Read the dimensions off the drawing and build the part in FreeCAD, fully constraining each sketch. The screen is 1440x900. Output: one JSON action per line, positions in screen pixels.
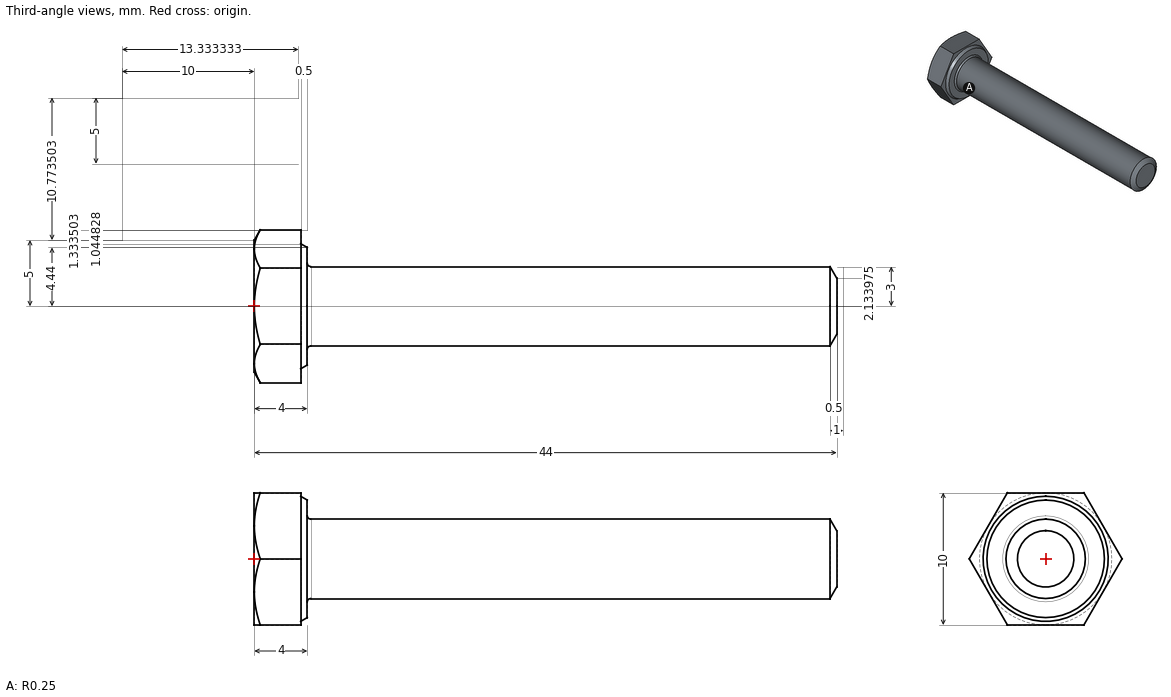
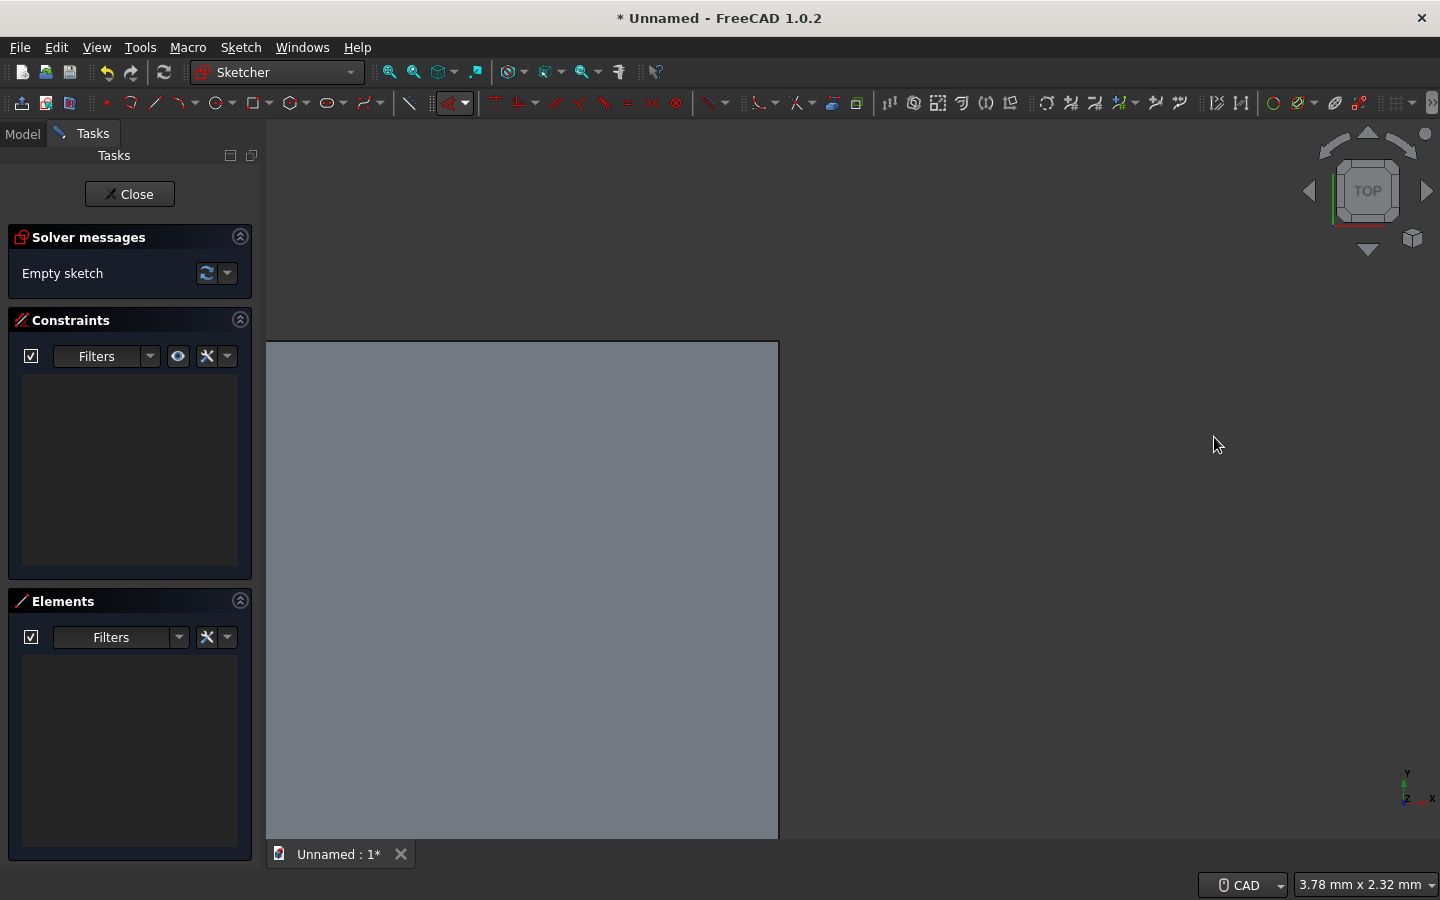
{"action": "scroll", "coordinate": [771, 470], "scroll_direction": "up", "scroll_amount": 3}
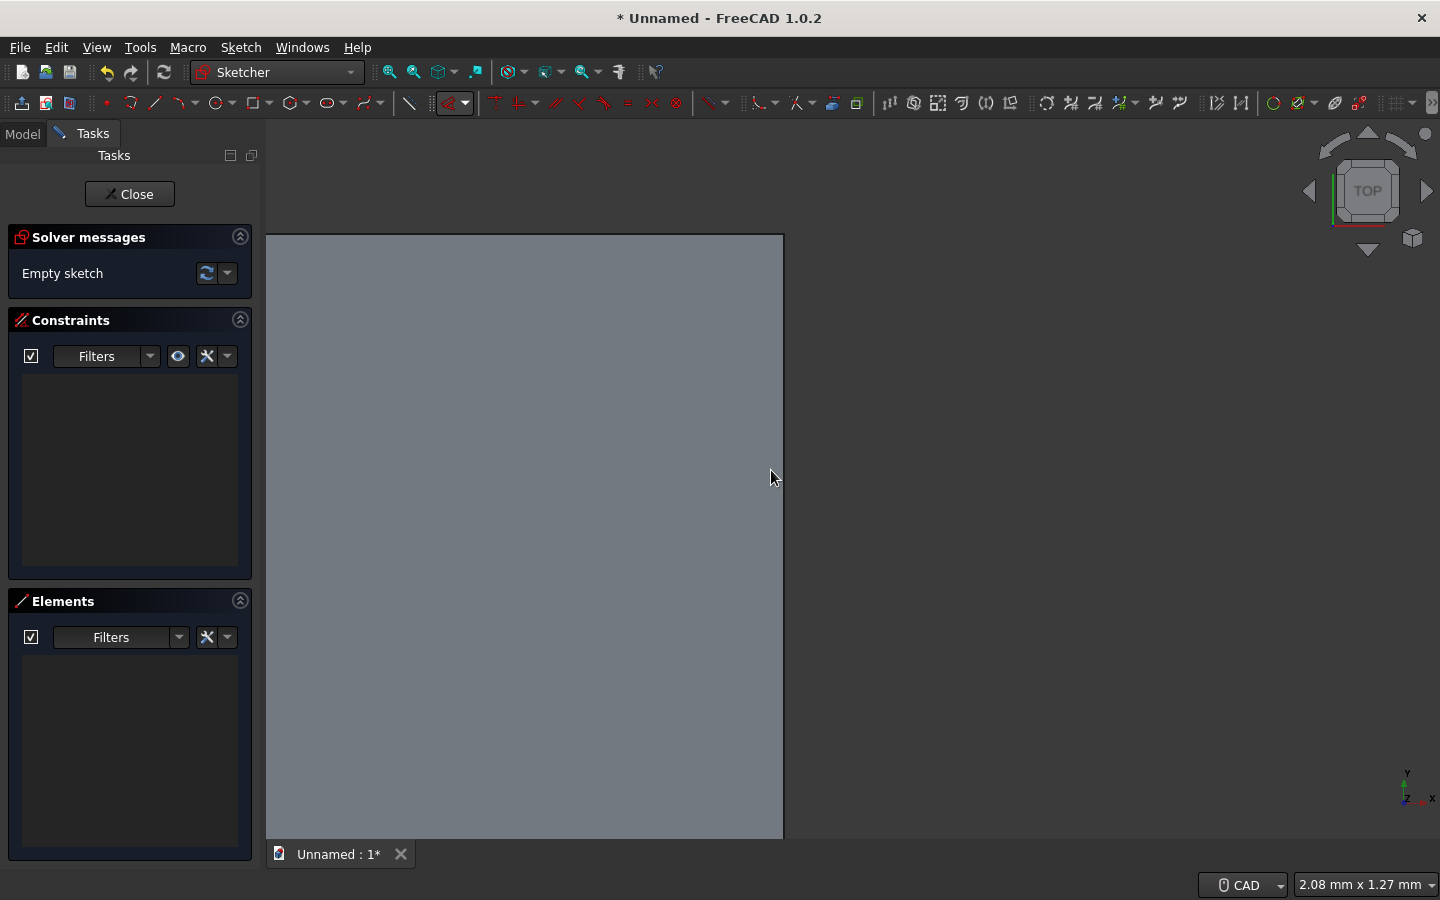
{"action": "left_click", "coordinate": [132, 104]}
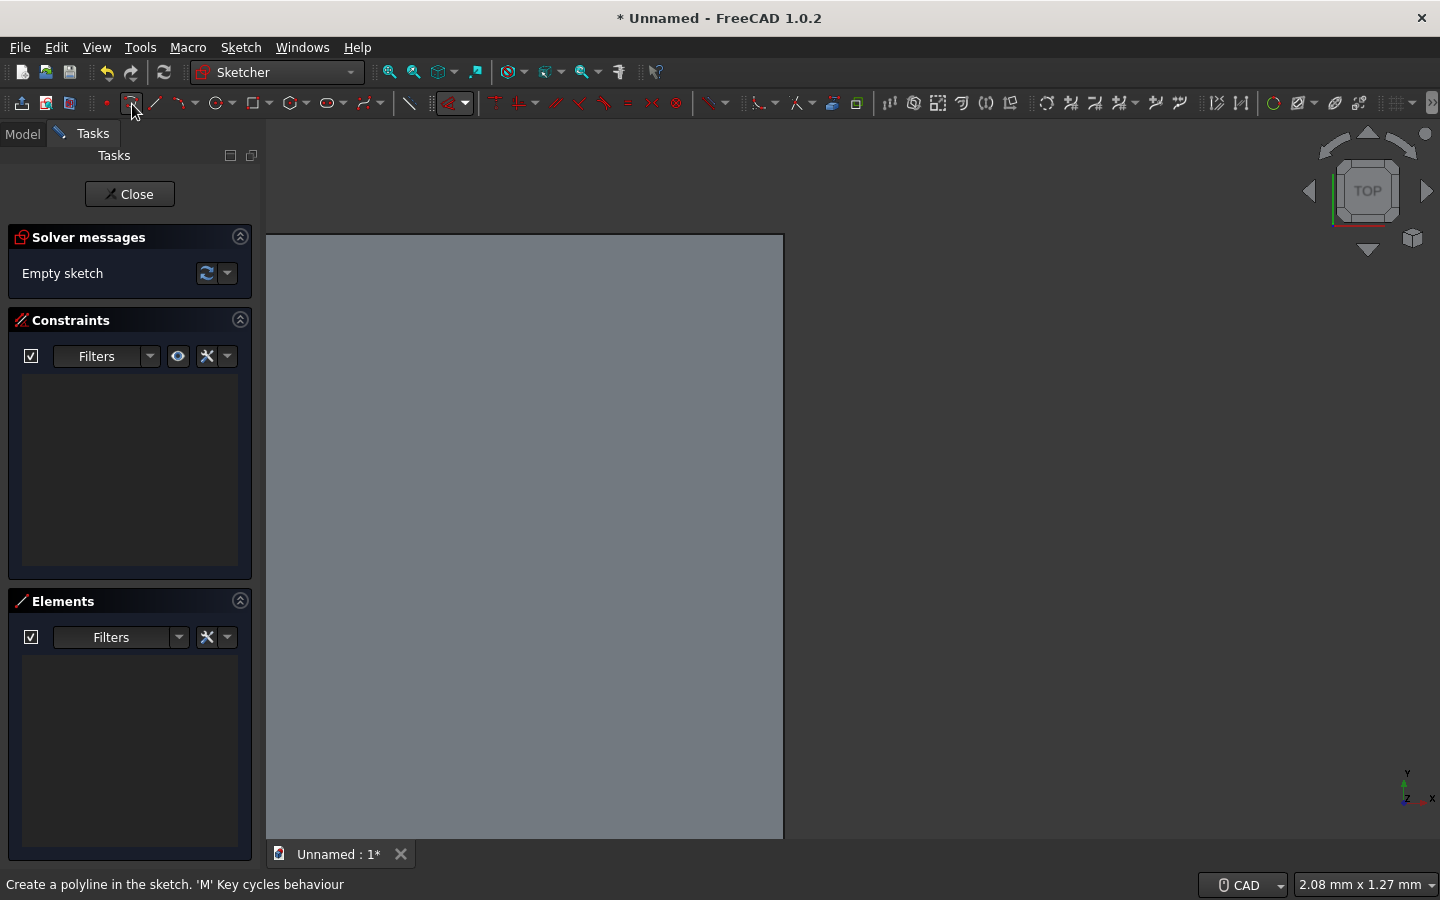
{"action": "left_click", "coordinate": [502, 234]}
{"action": "left_click", "coordinate": [784, 724]}
{"action": "left_click", "coordinate": [1067, 234]}
{"action": "left_click", "coordinate": [502, 235]}
{"action": "key", "text": "Escape"}
{"action": "key", "text": "Escape"}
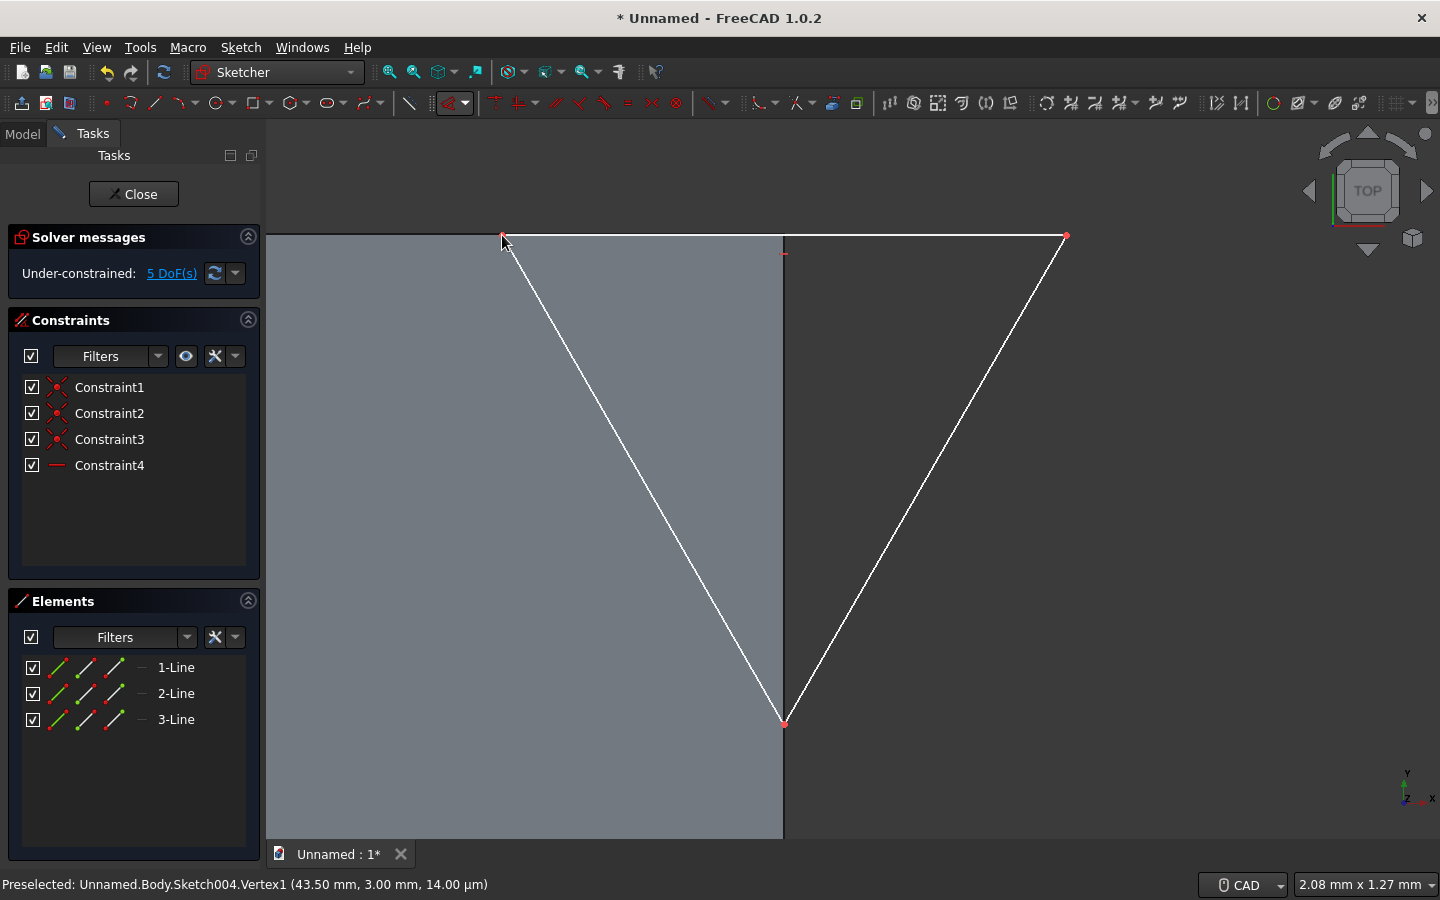
{"action": "left_click", "coordinate": [898, 235]}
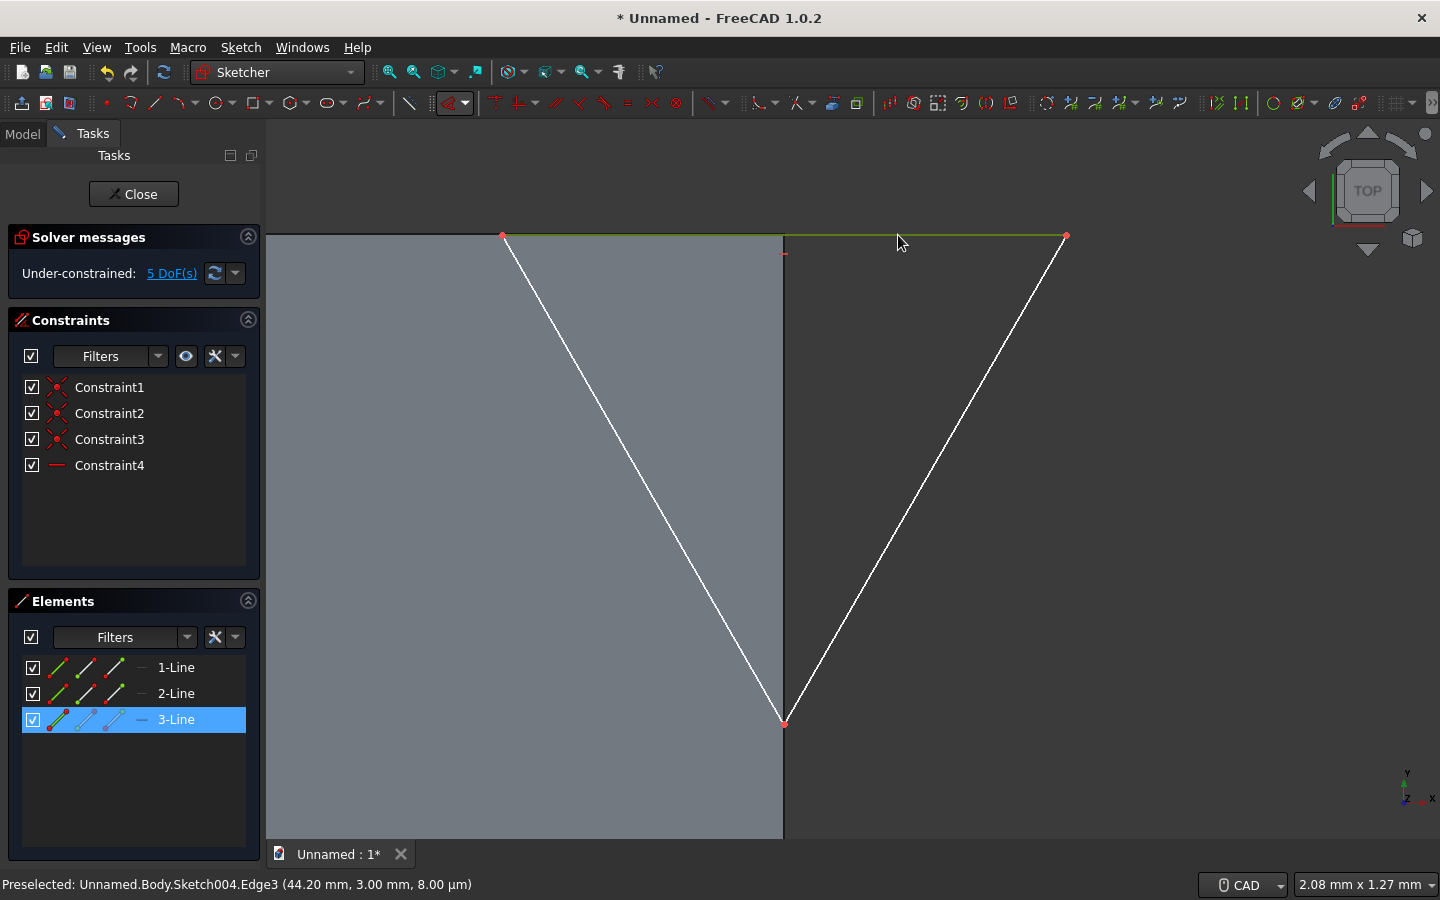
{"action": "key", "text": "l"}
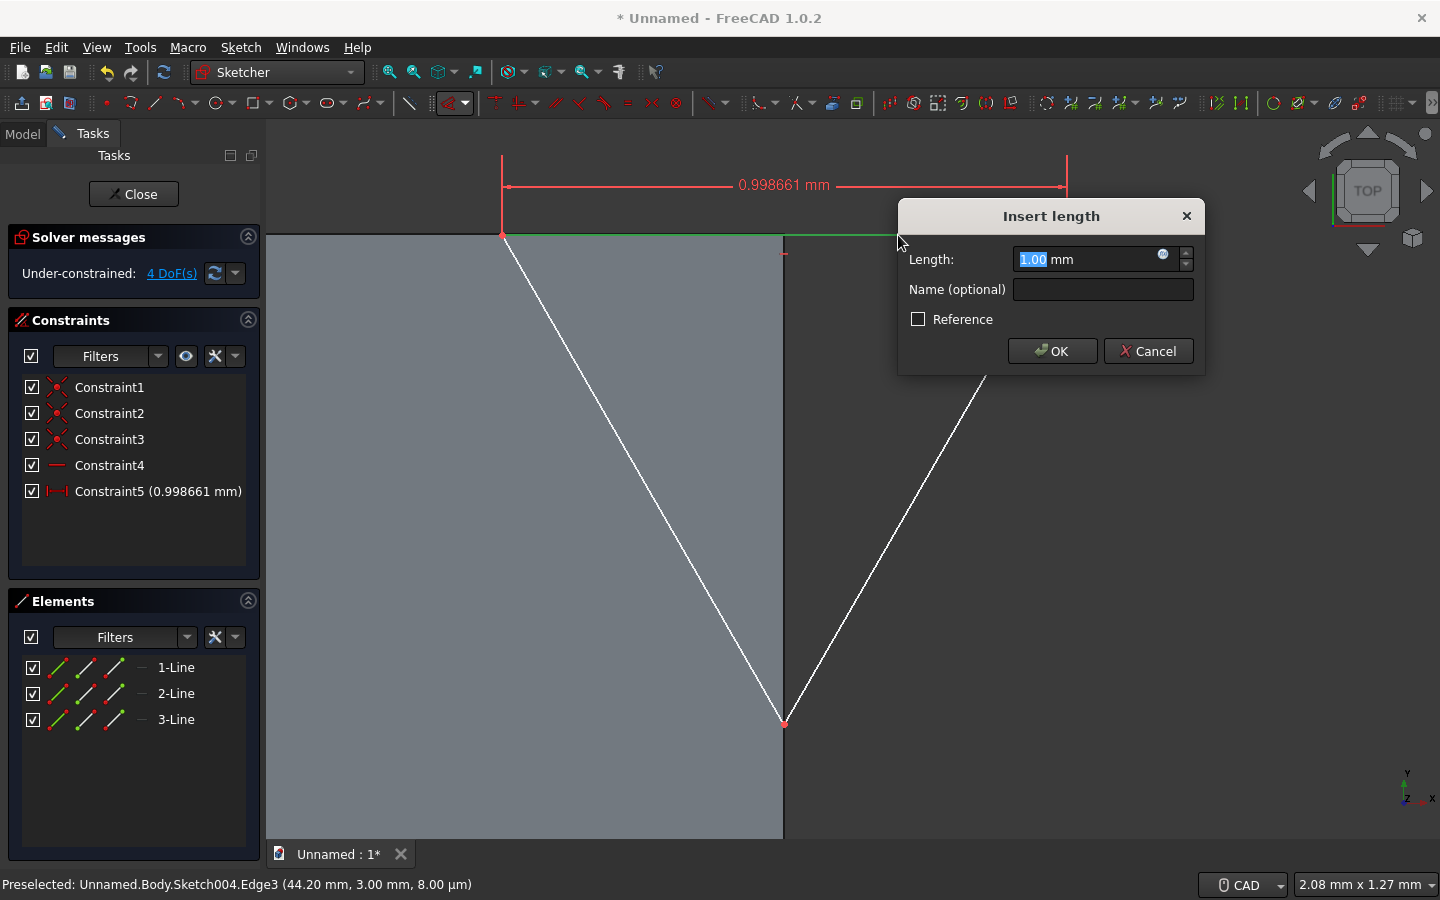
{"action": "type", "text": "1"}
{"action": "key", "text": "Return"}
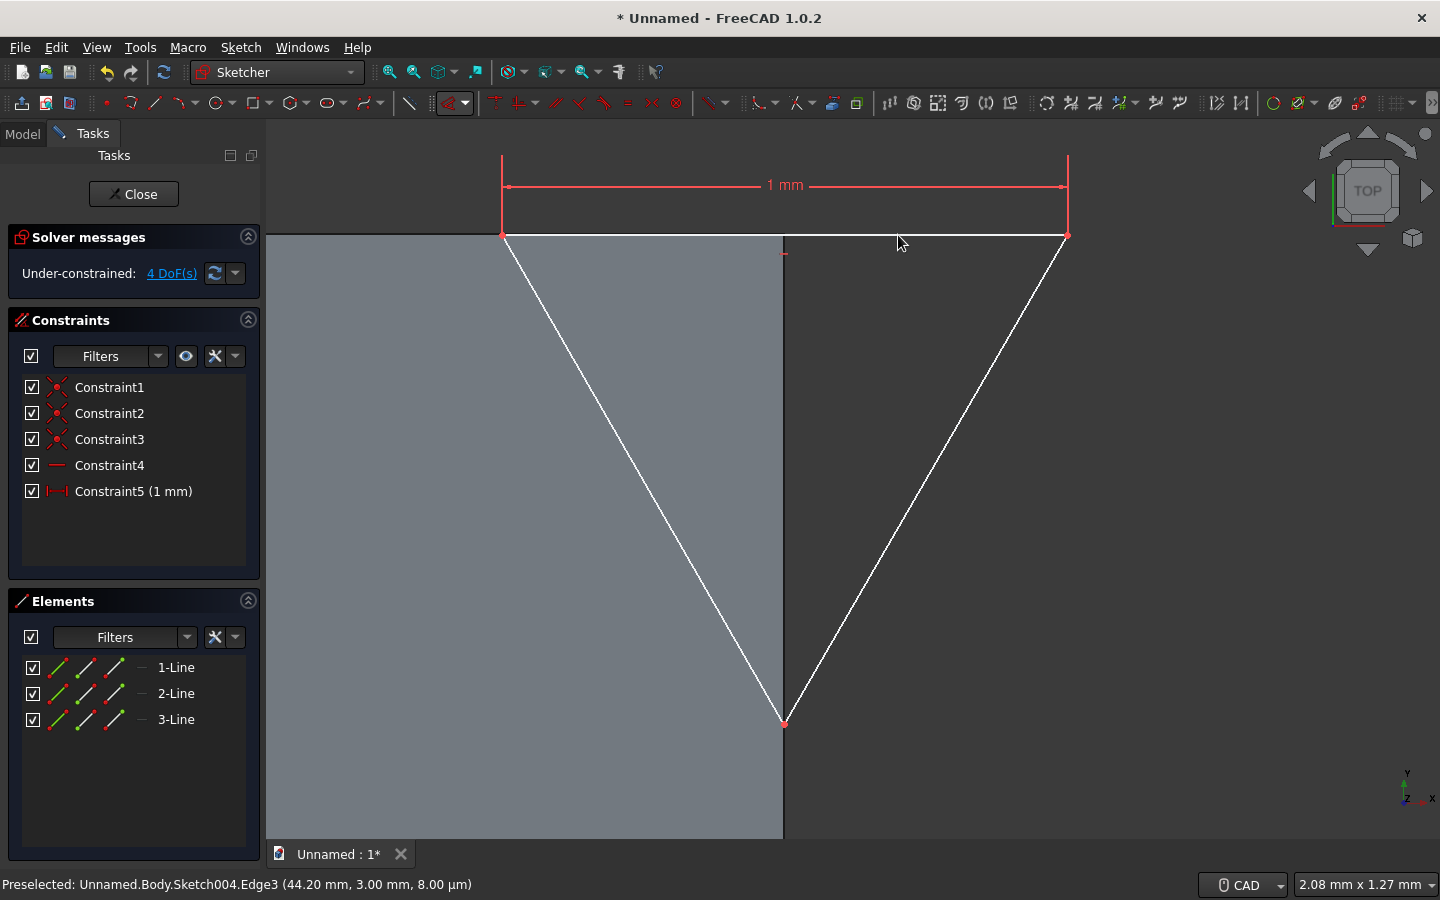
{"action": "left_click", "coordinate": [502, 235]}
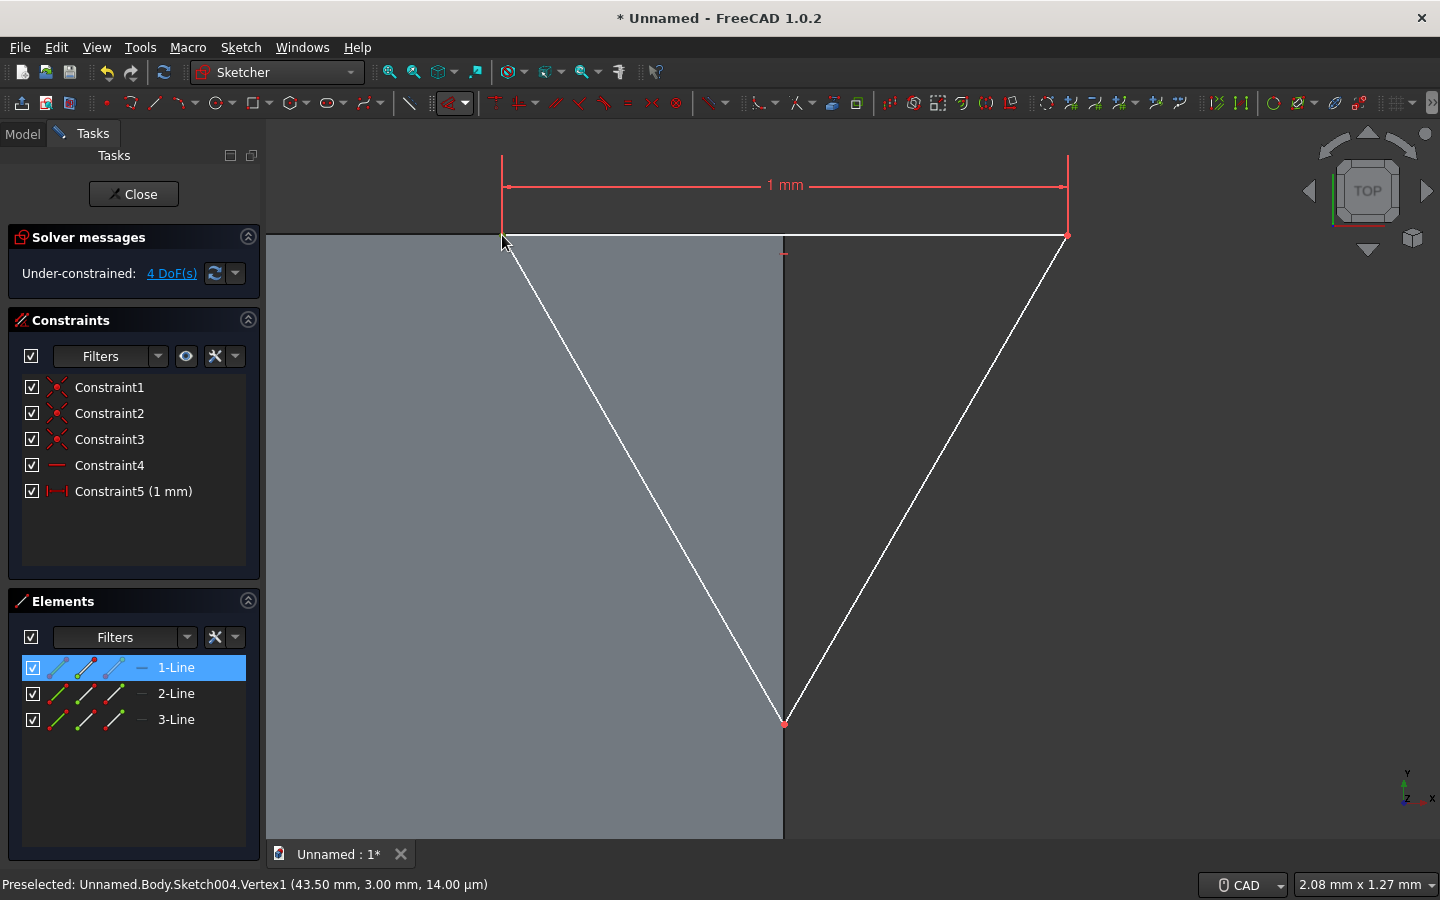
{"action": "left_click", "coordinate": [468, 104]}